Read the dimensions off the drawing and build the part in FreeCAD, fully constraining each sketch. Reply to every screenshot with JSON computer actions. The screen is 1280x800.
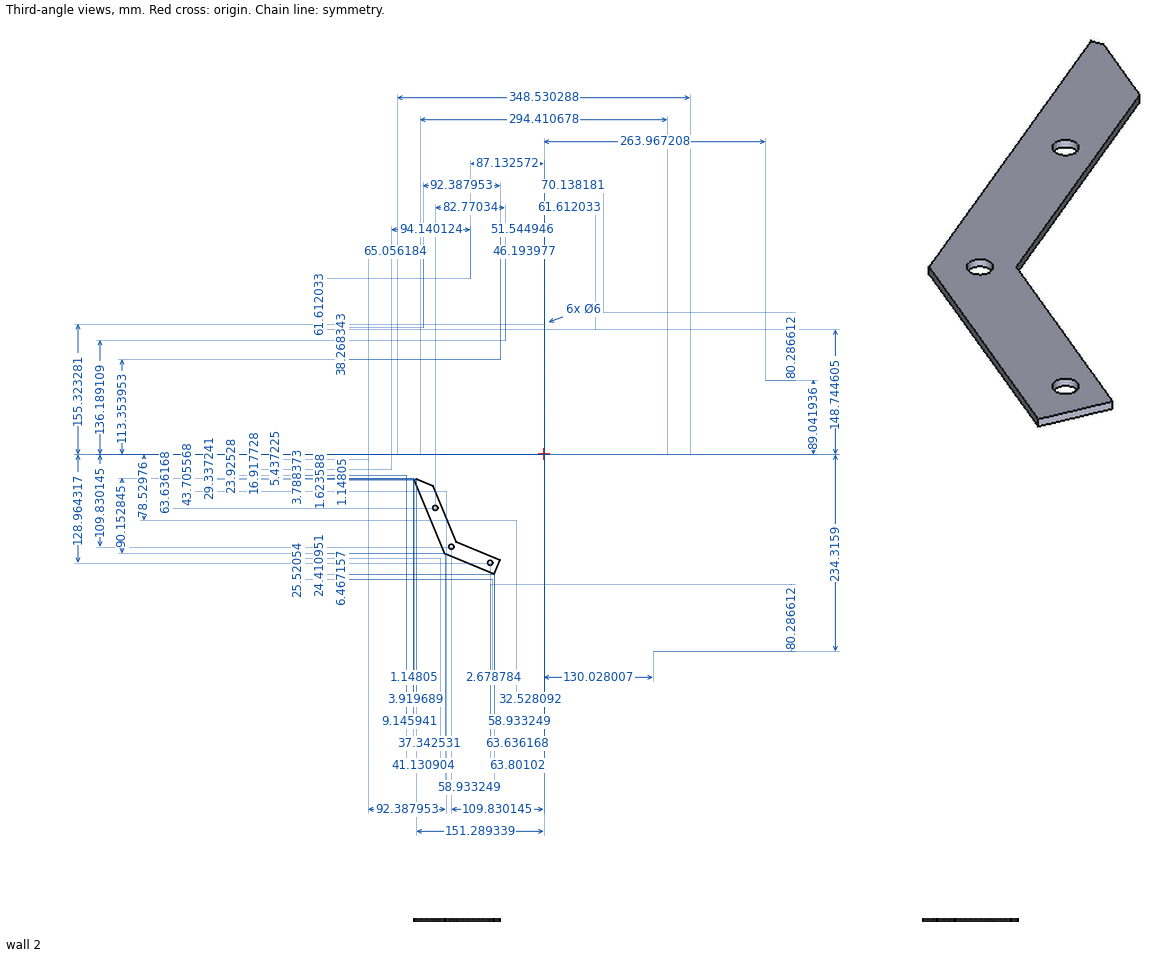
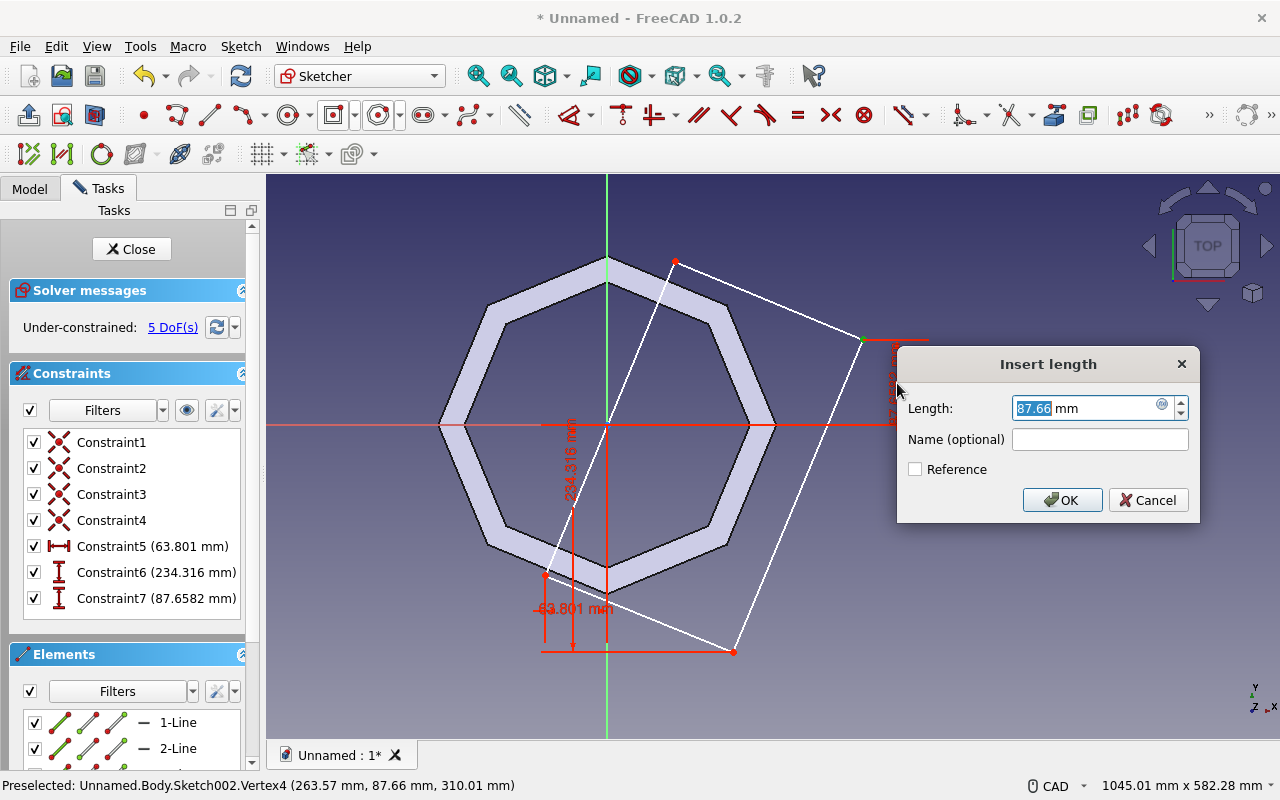
{"action": "type", "text": "89.041936"}
{"action": "key", "text": "Return"}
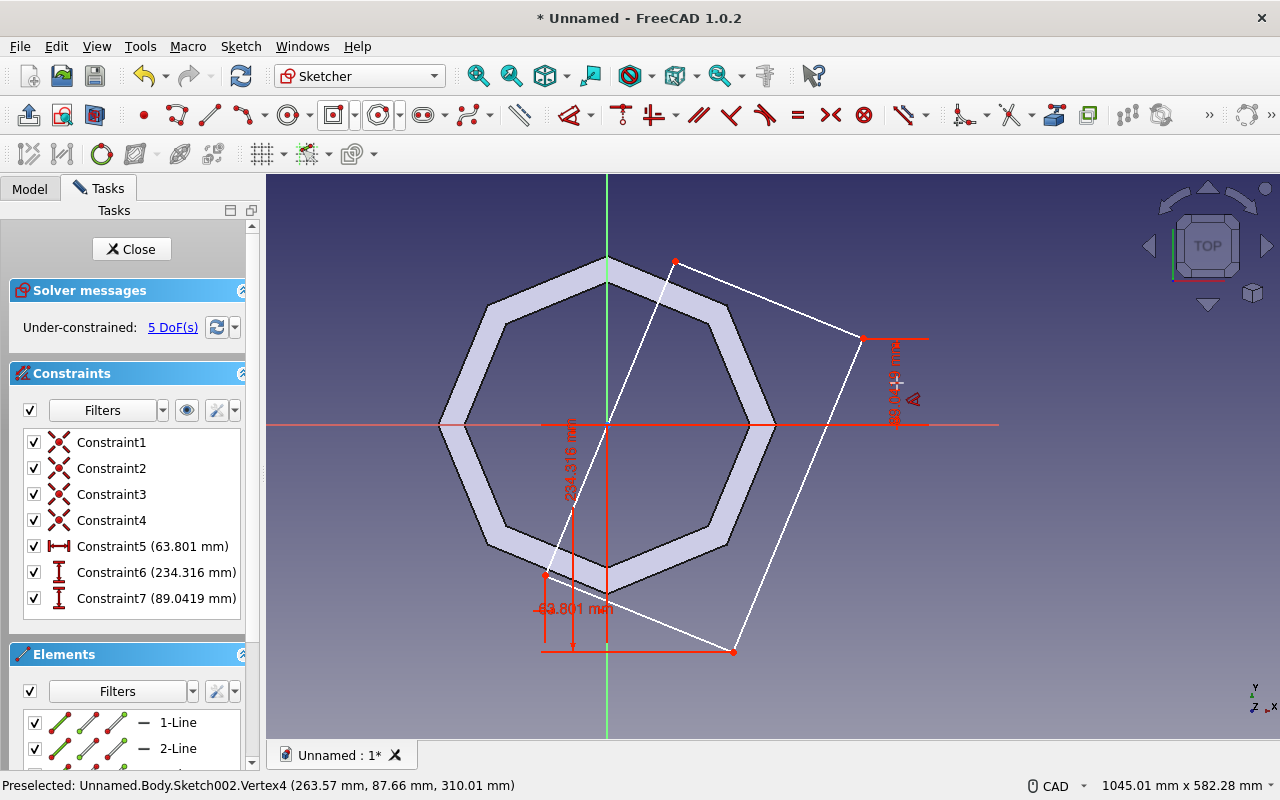
{"action": "left_click", "coordinate": [675, 262]}
{"action": "left_click", "coordinate": [641, 228]}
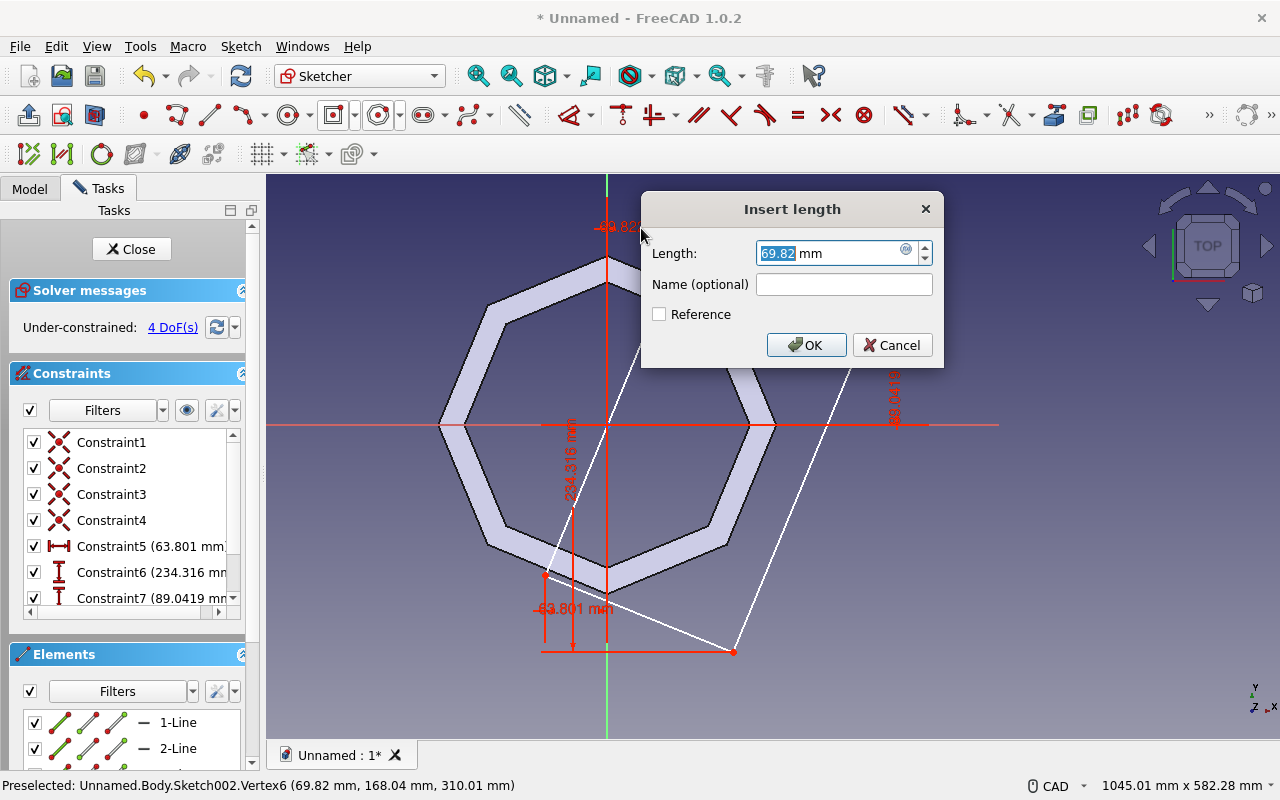
{"action": "type", "text": "70.138181"}
{"action": "key", "text": "Return"}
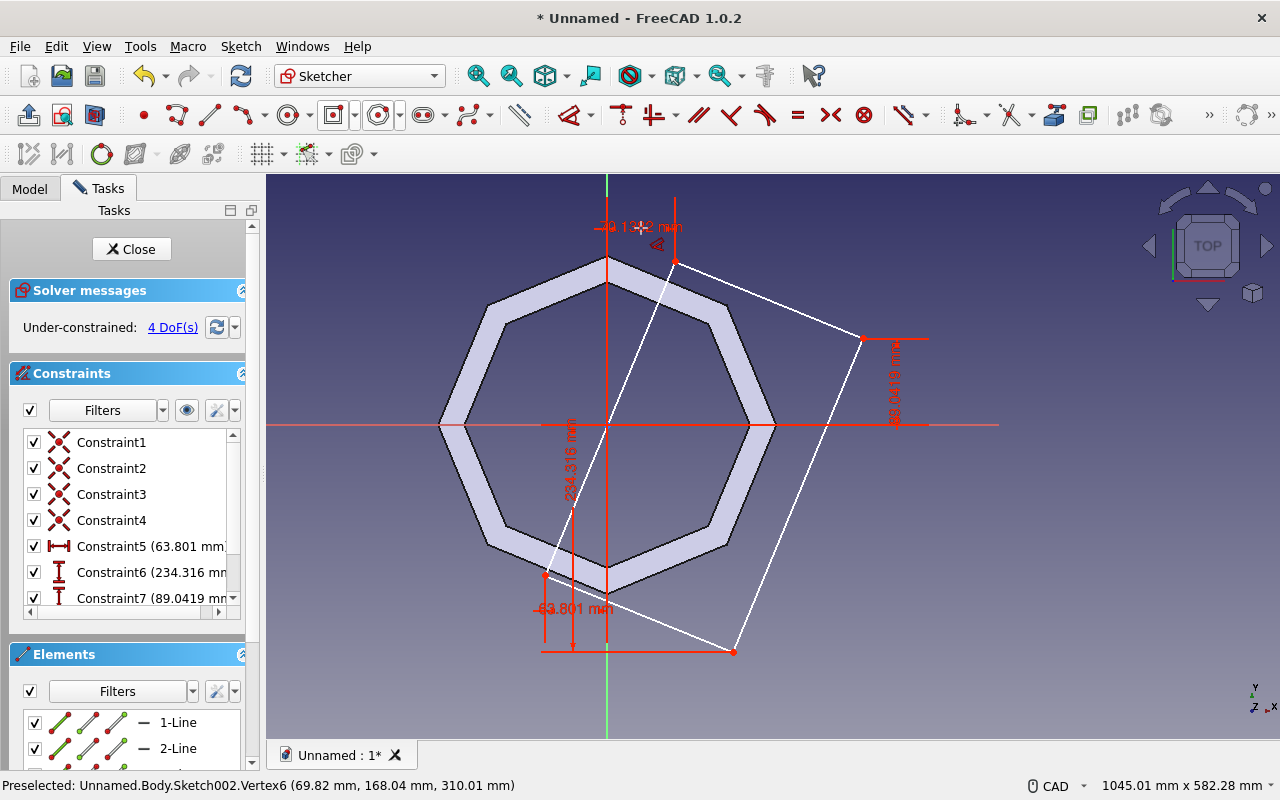
{"action": "left_click", "coordinate": [677, 629]}
{"action": "left_click", "coordinate": [511, 632]}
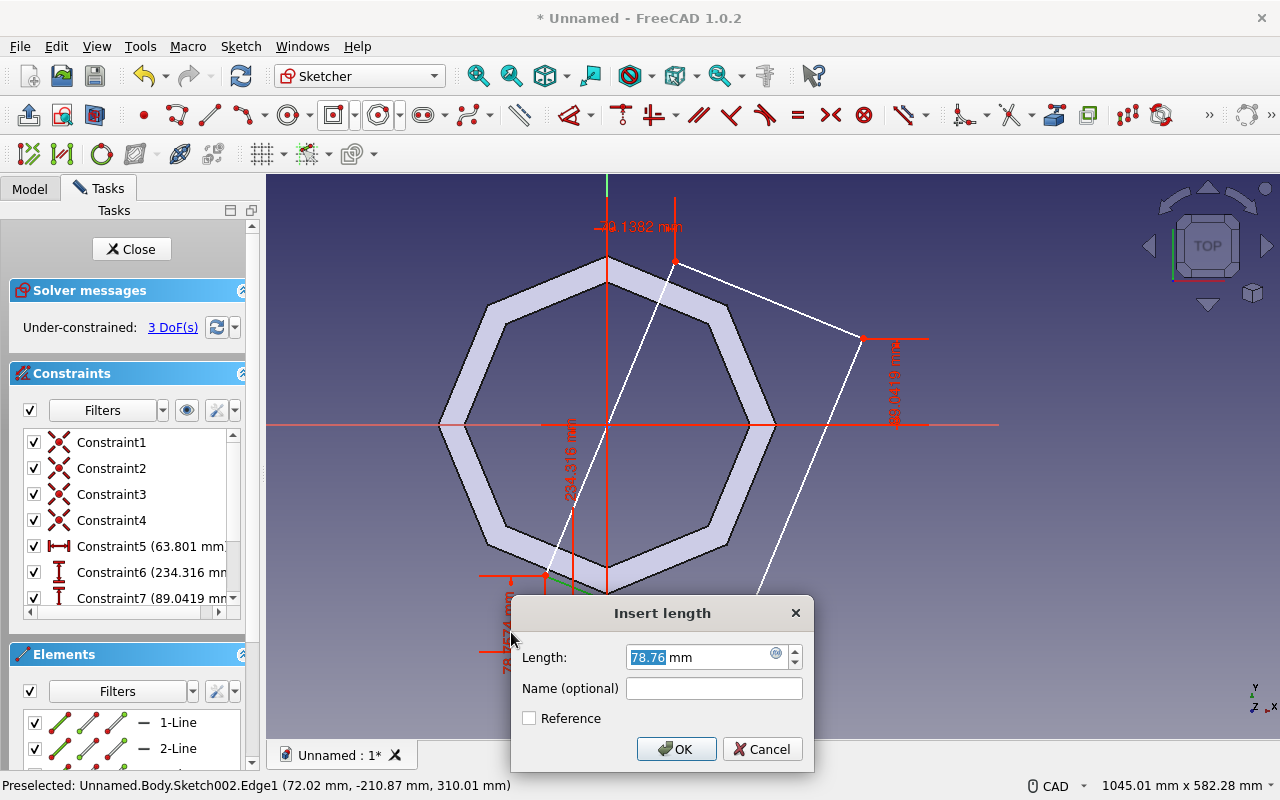
{"action": "type", "text": "80.286612"}
{"action": "key", "text": "Return"}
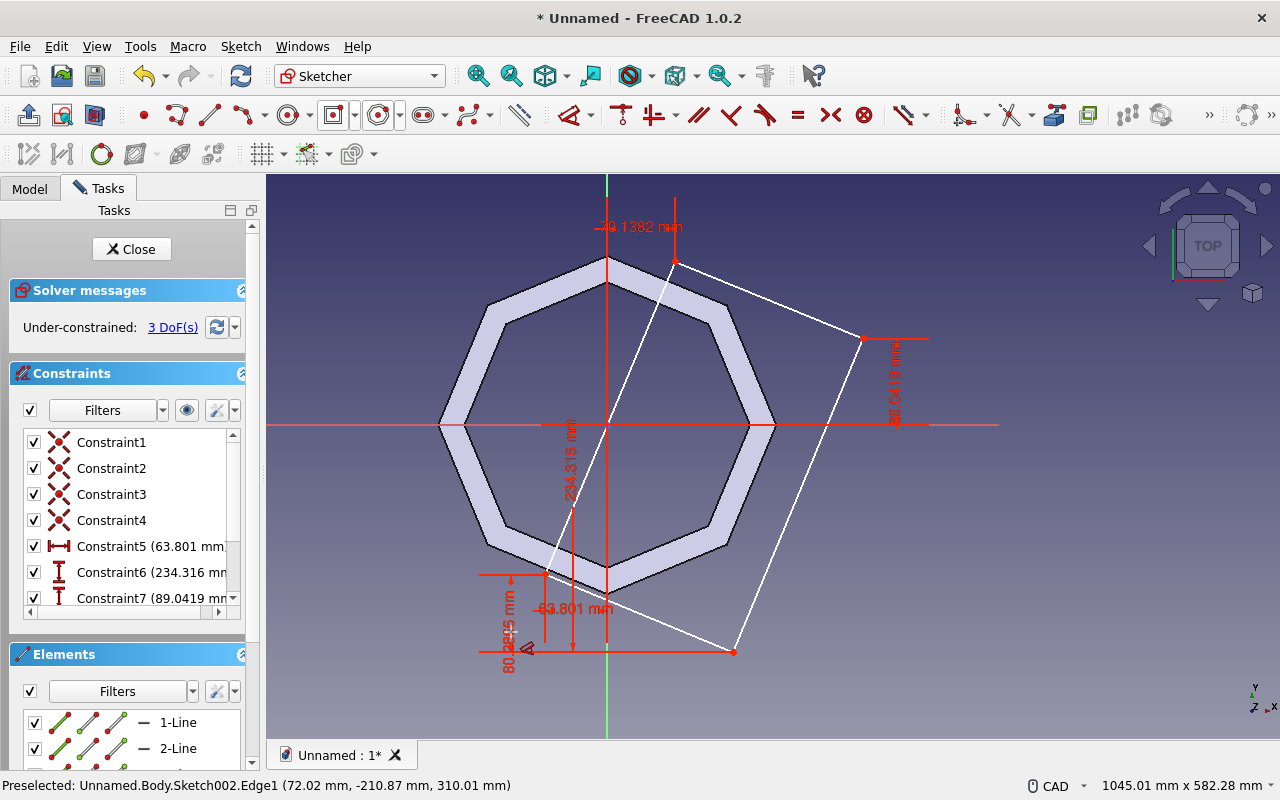
{"action": "left_click", "coordinate": [807, 316]}
{"action": "left_click", "coordinate": [897, 300]}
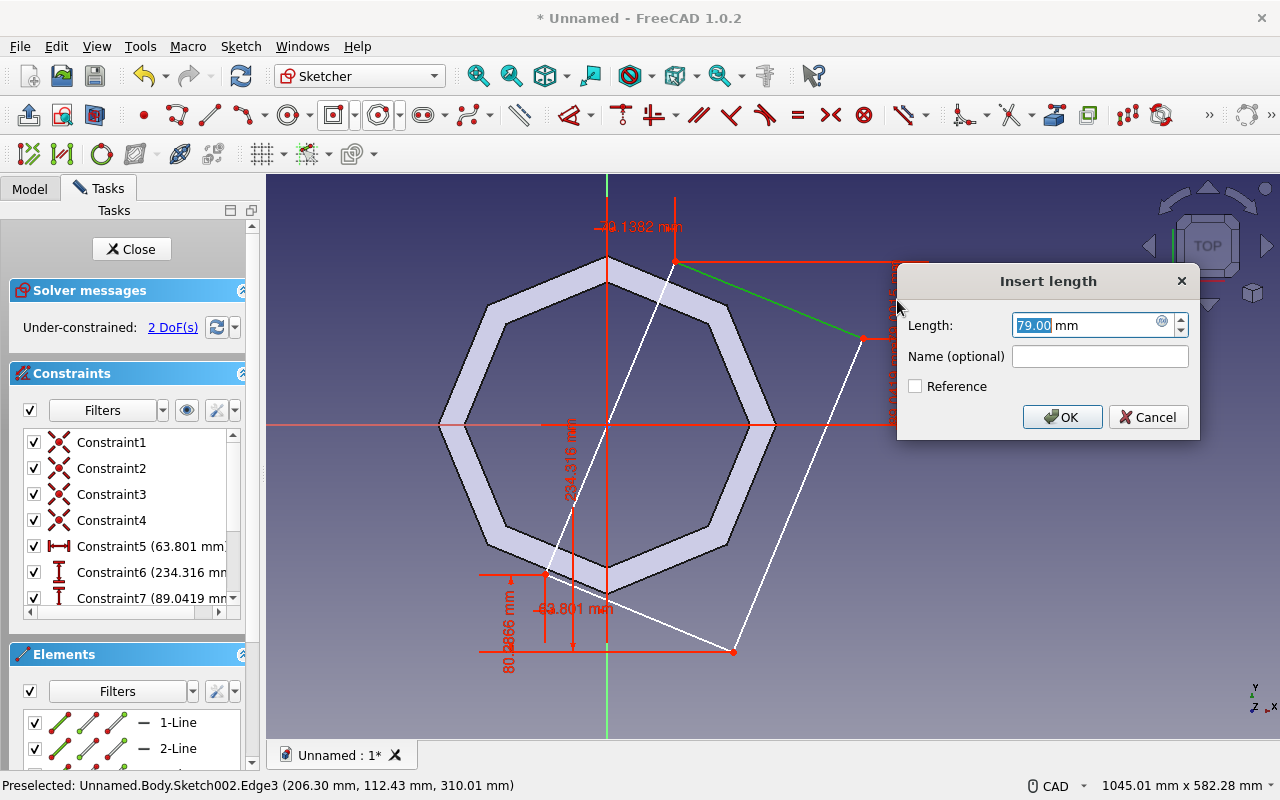
{"action": "type", "text": "80.286612"}
{"action": "key", "text": "Return"}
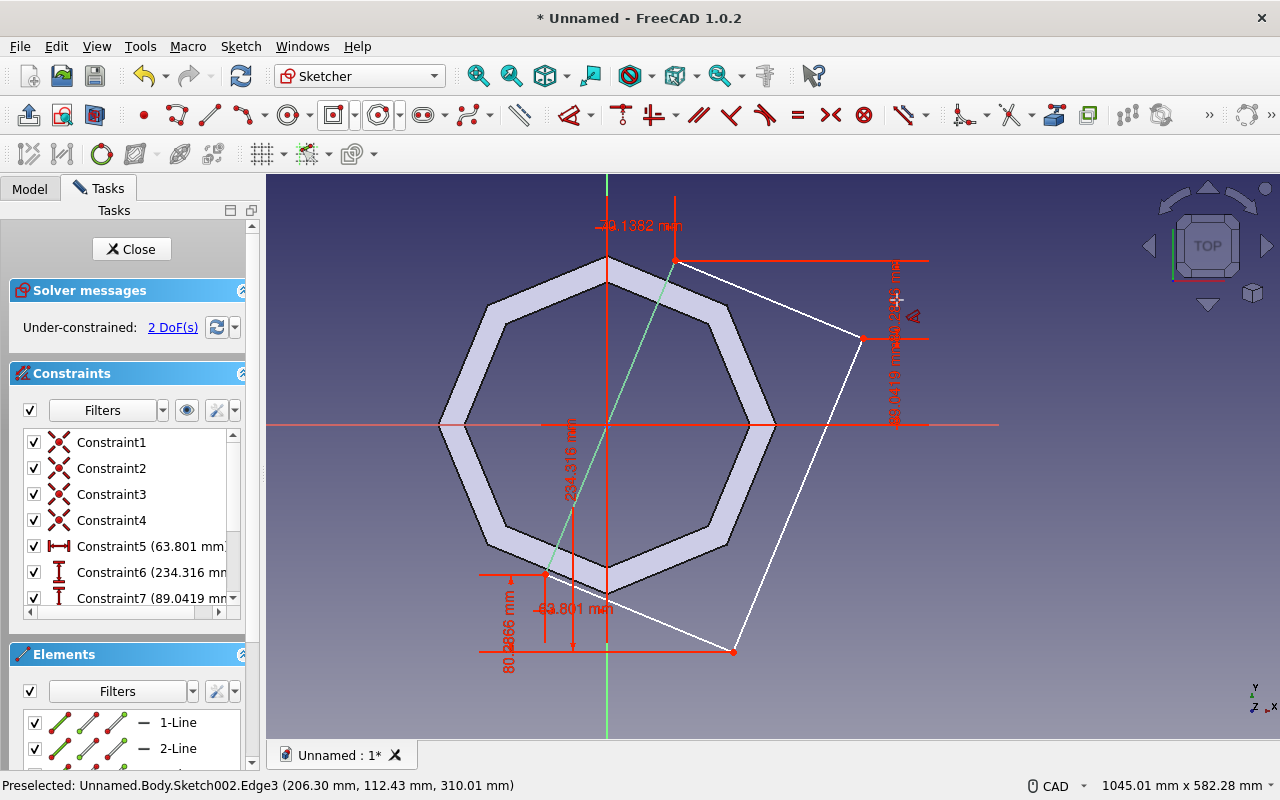
{"action": "left_click", "coordinate": [733, 652]}
{"action": "left_click", "coordinate": [670, 686]}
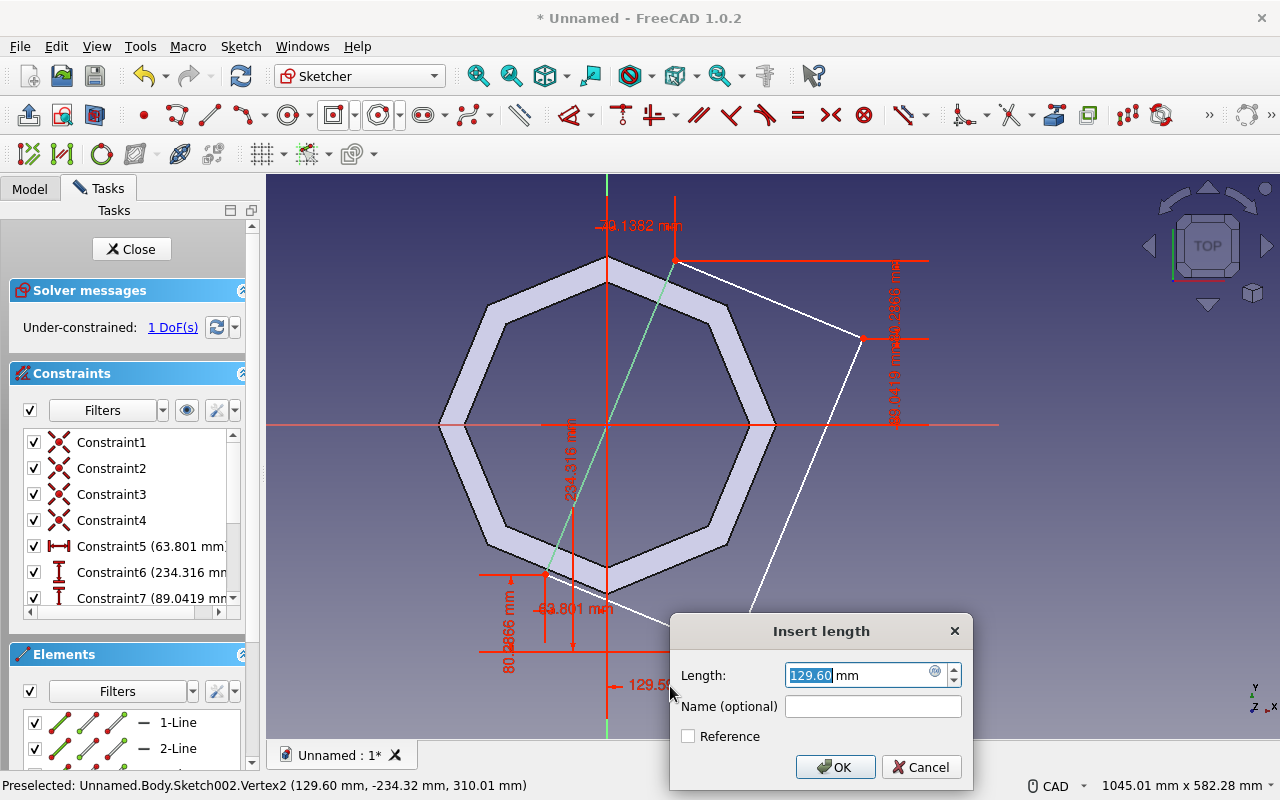
{"action": "type", "text": "130.028007"}
{"action": "key", "text": "Return"}